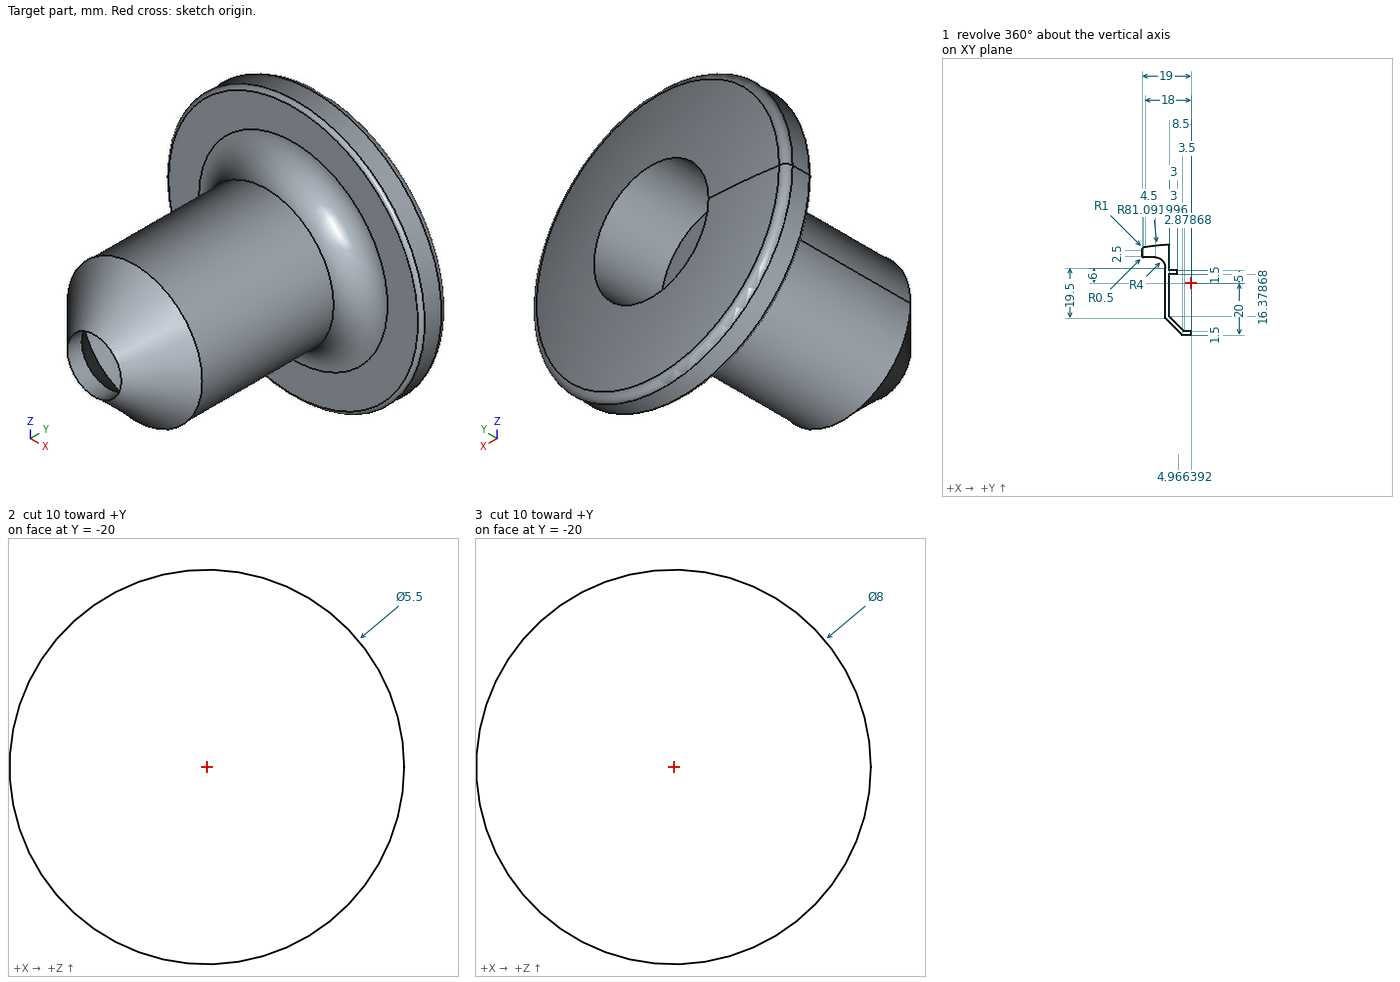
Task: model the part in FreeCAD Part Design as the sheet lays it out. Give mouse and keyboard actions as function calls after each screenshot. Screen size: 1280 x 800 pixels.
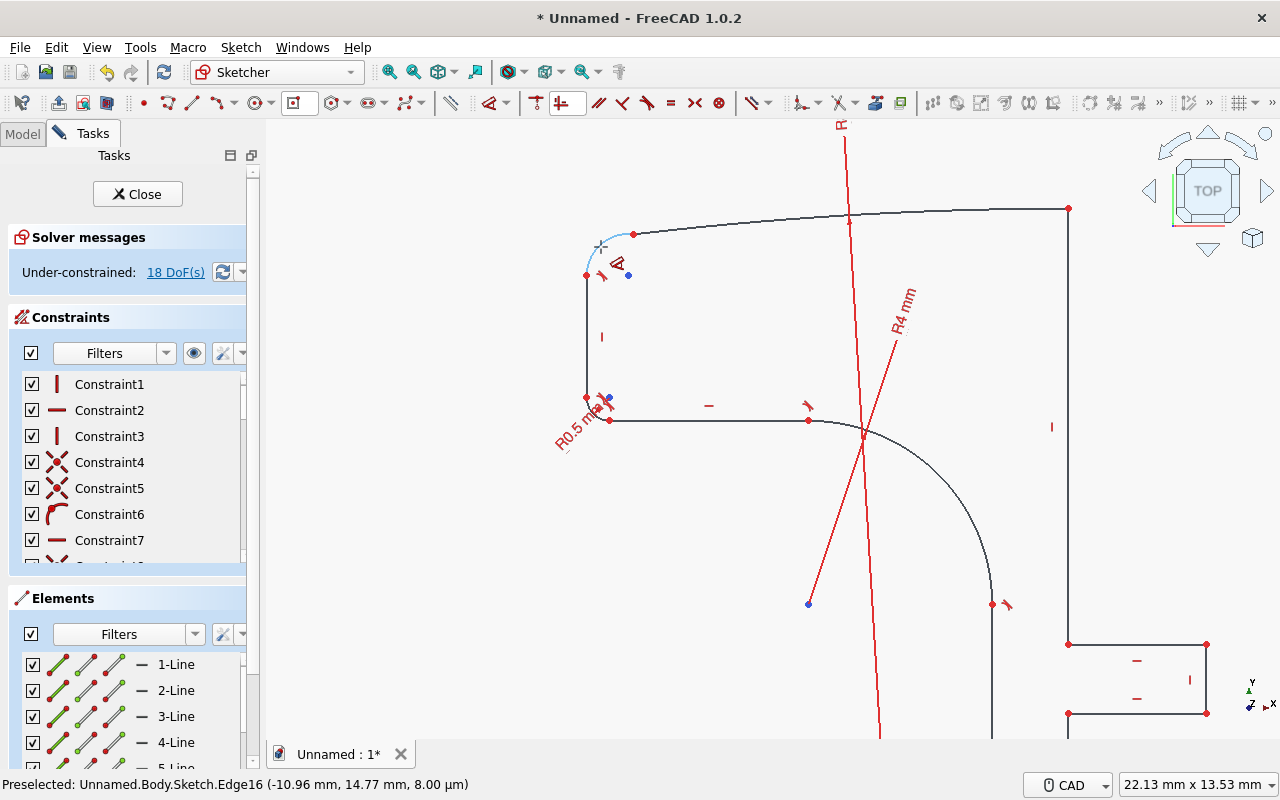
click(601, 244)
click(580, 220)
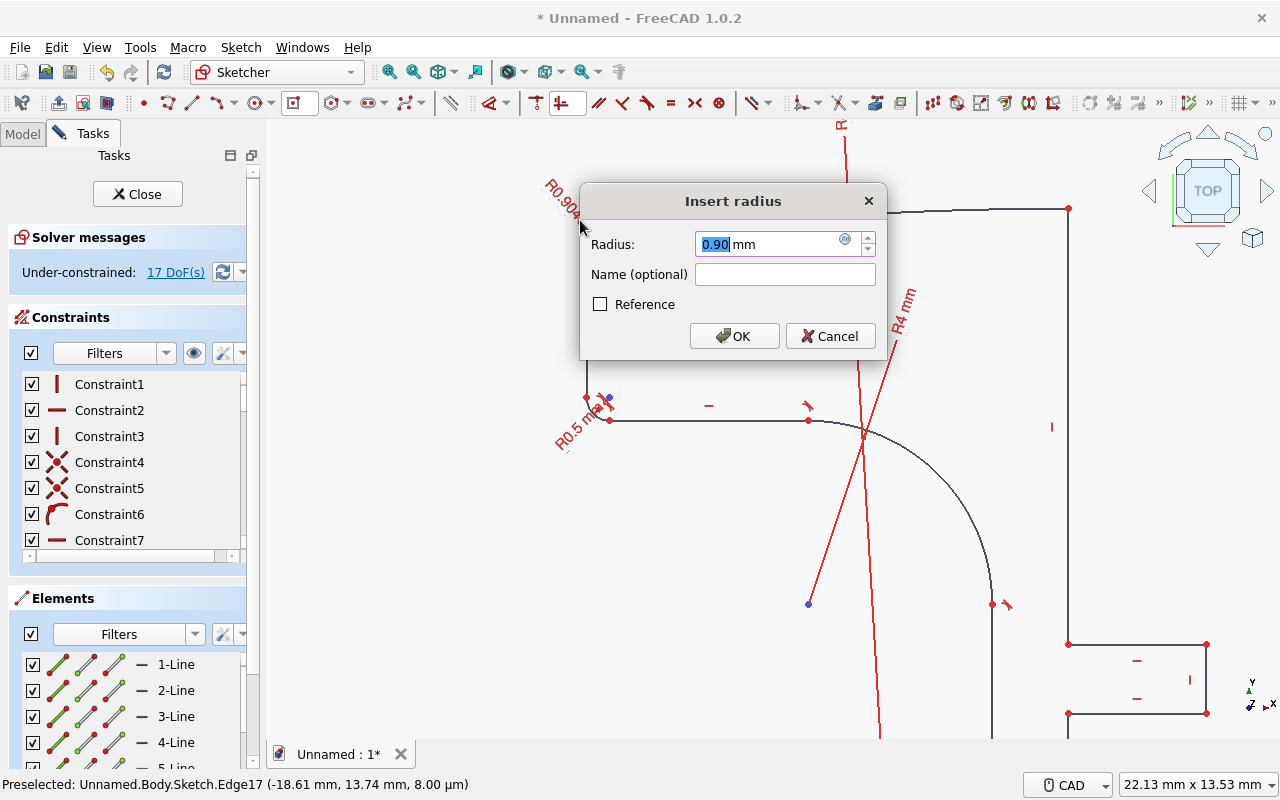
text(1)
key(Return)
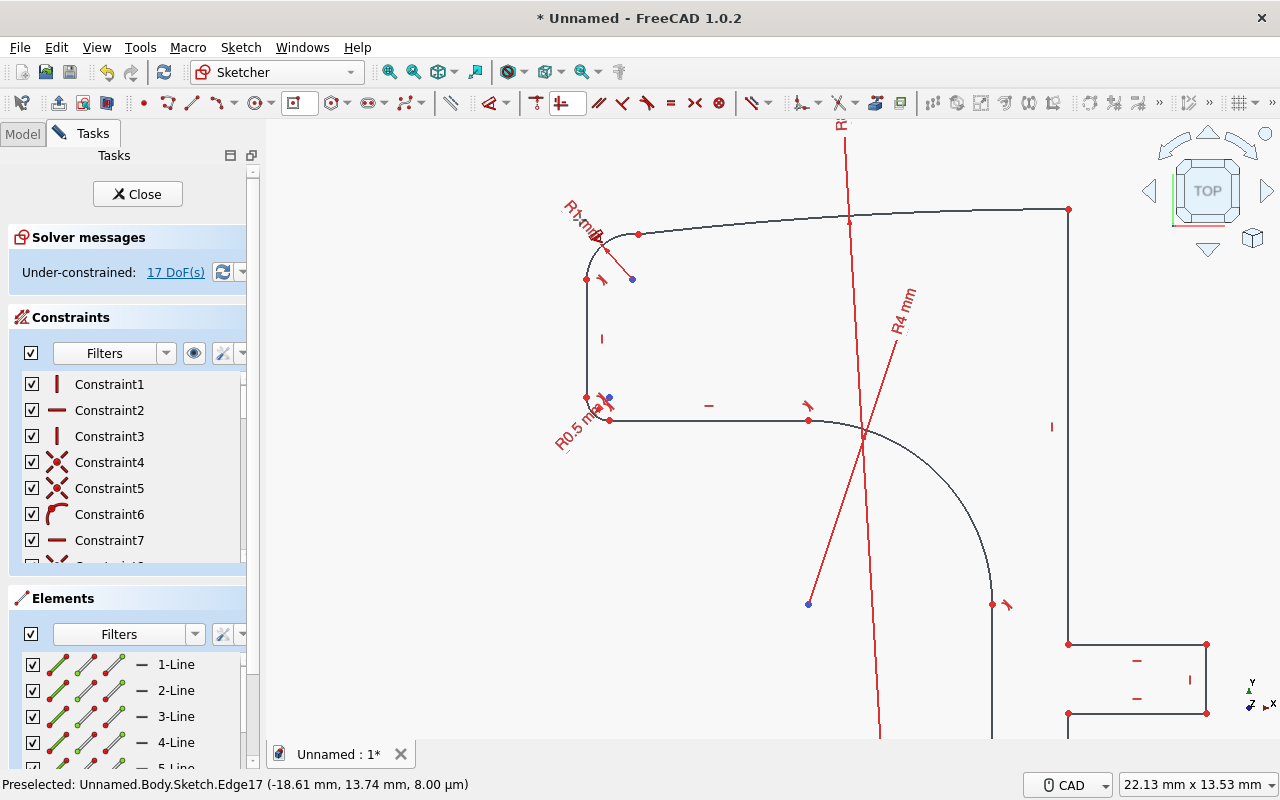
scroll(601, 247, down, 7)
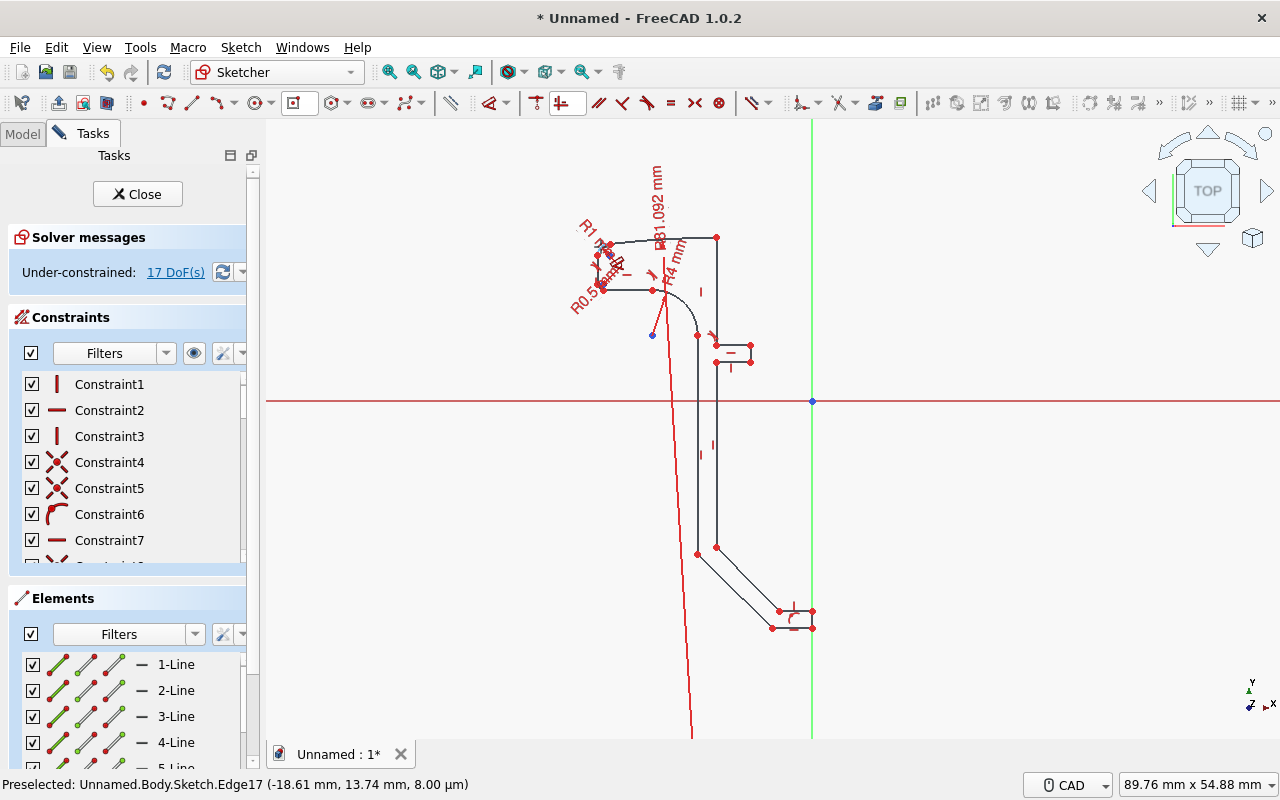
scroll(727, 362, up, 2)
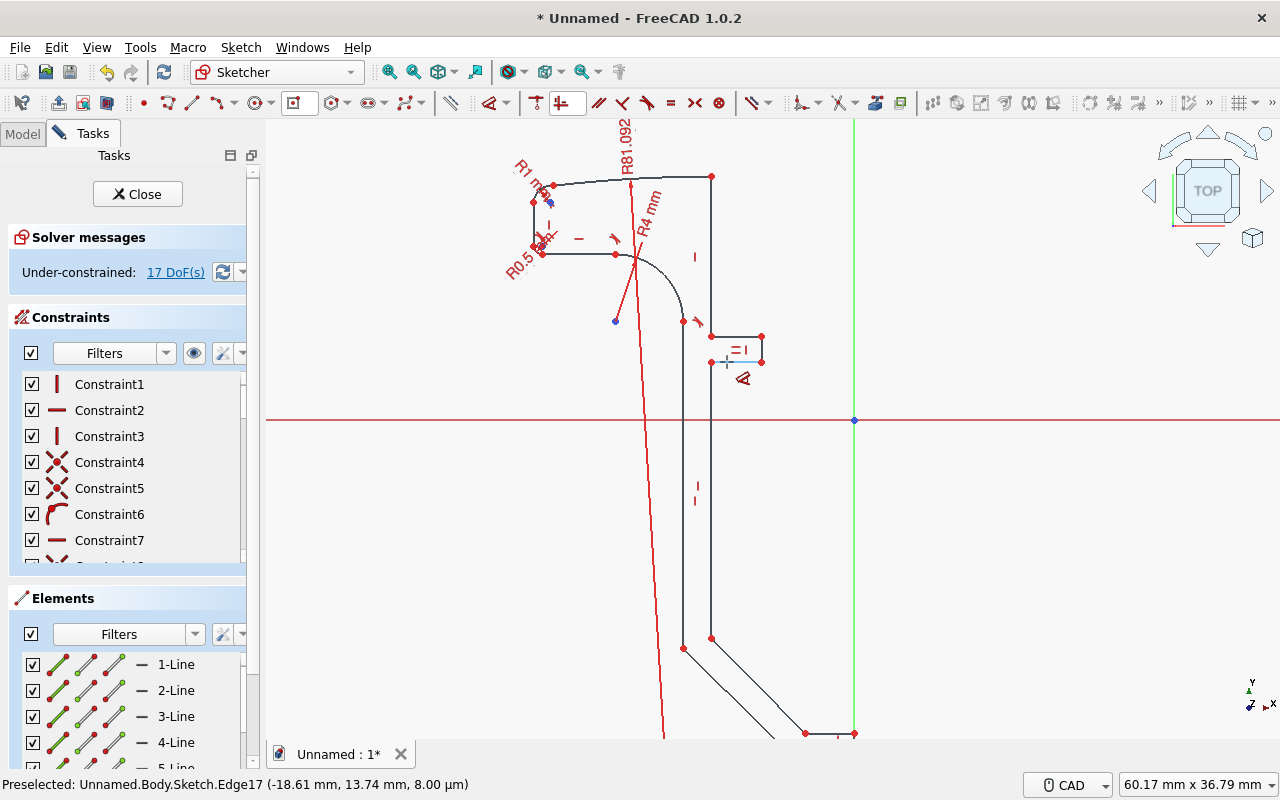
click(726, 362)
click(737, 396)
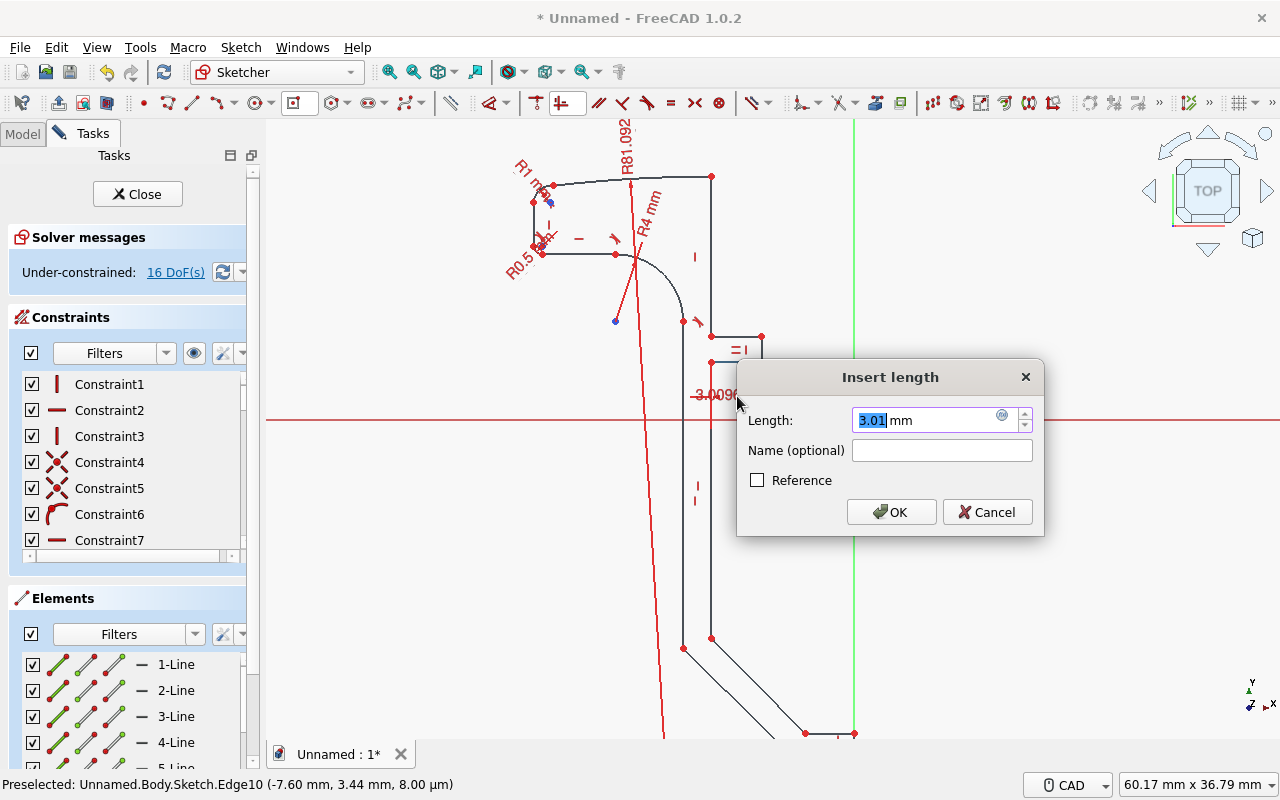
text(3)
key(Return)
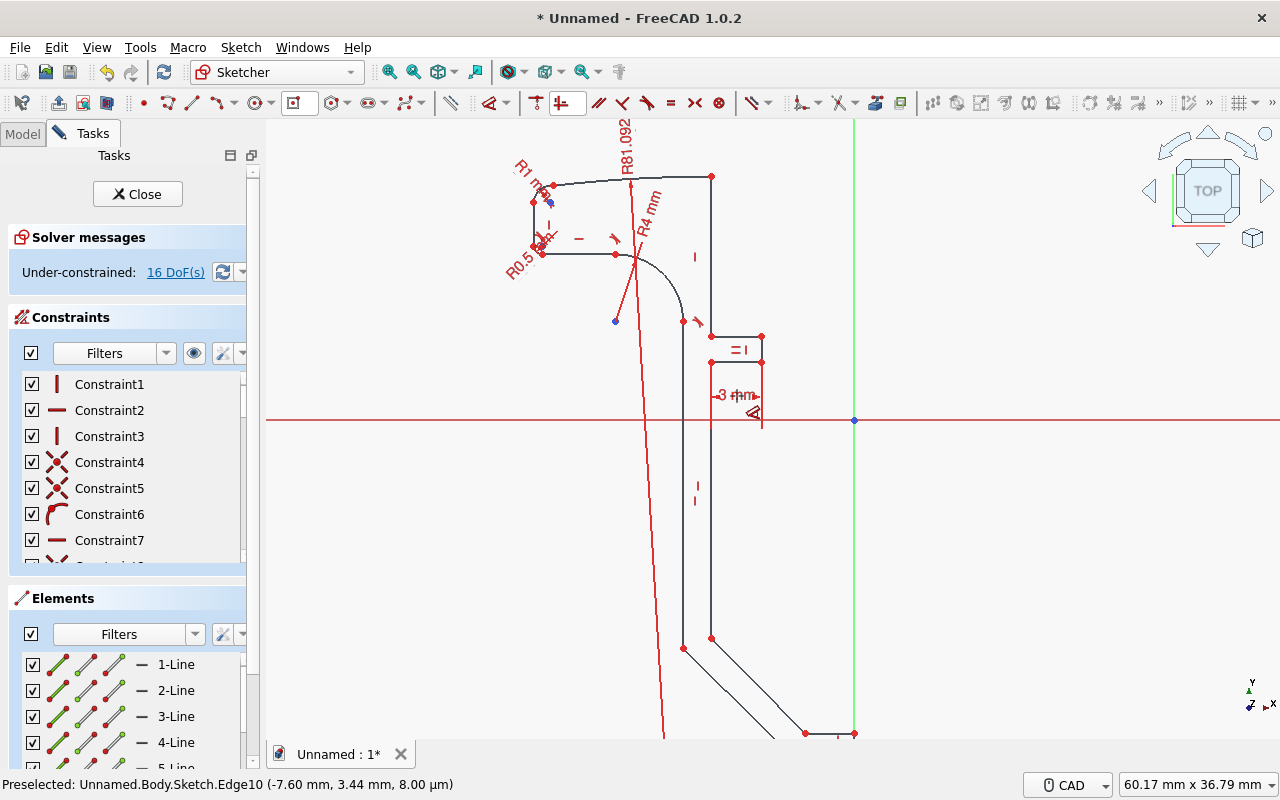
click(747, 337)
click(736, 303)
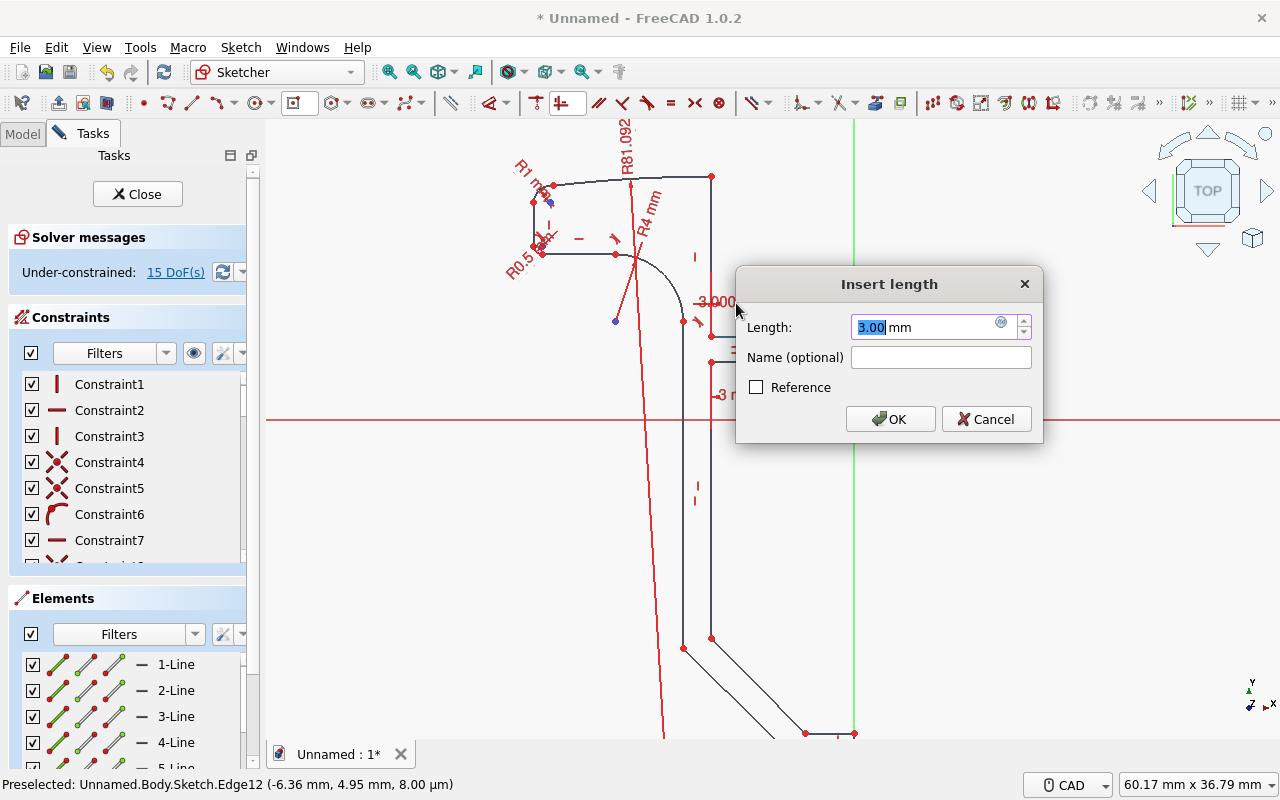
text(3)
key(Return)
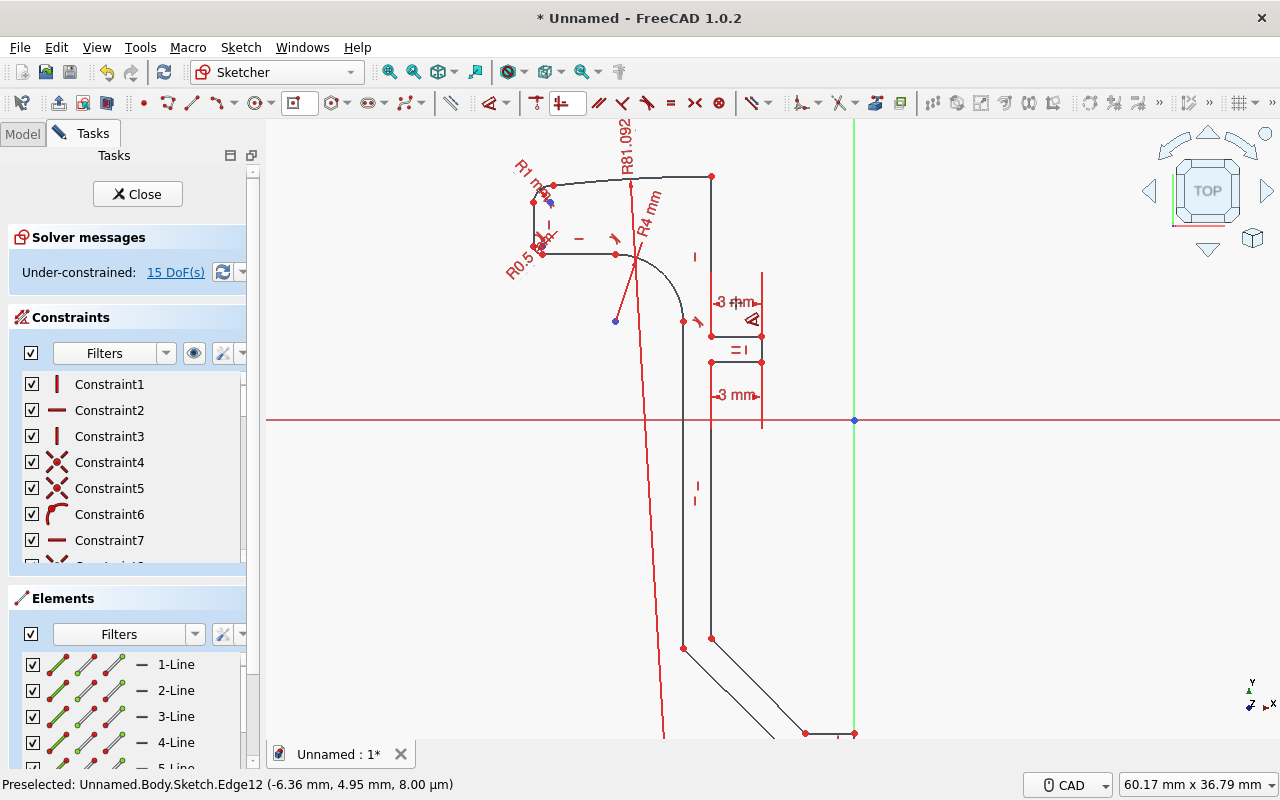
click(683, 322)
click(888, 371)